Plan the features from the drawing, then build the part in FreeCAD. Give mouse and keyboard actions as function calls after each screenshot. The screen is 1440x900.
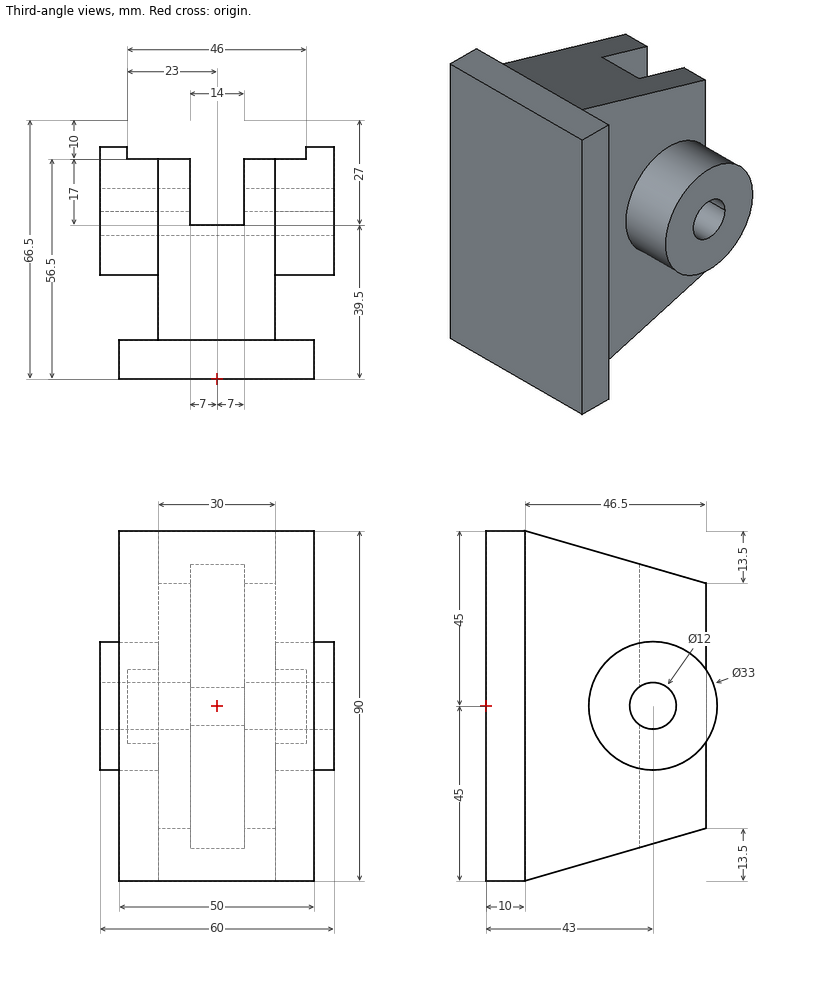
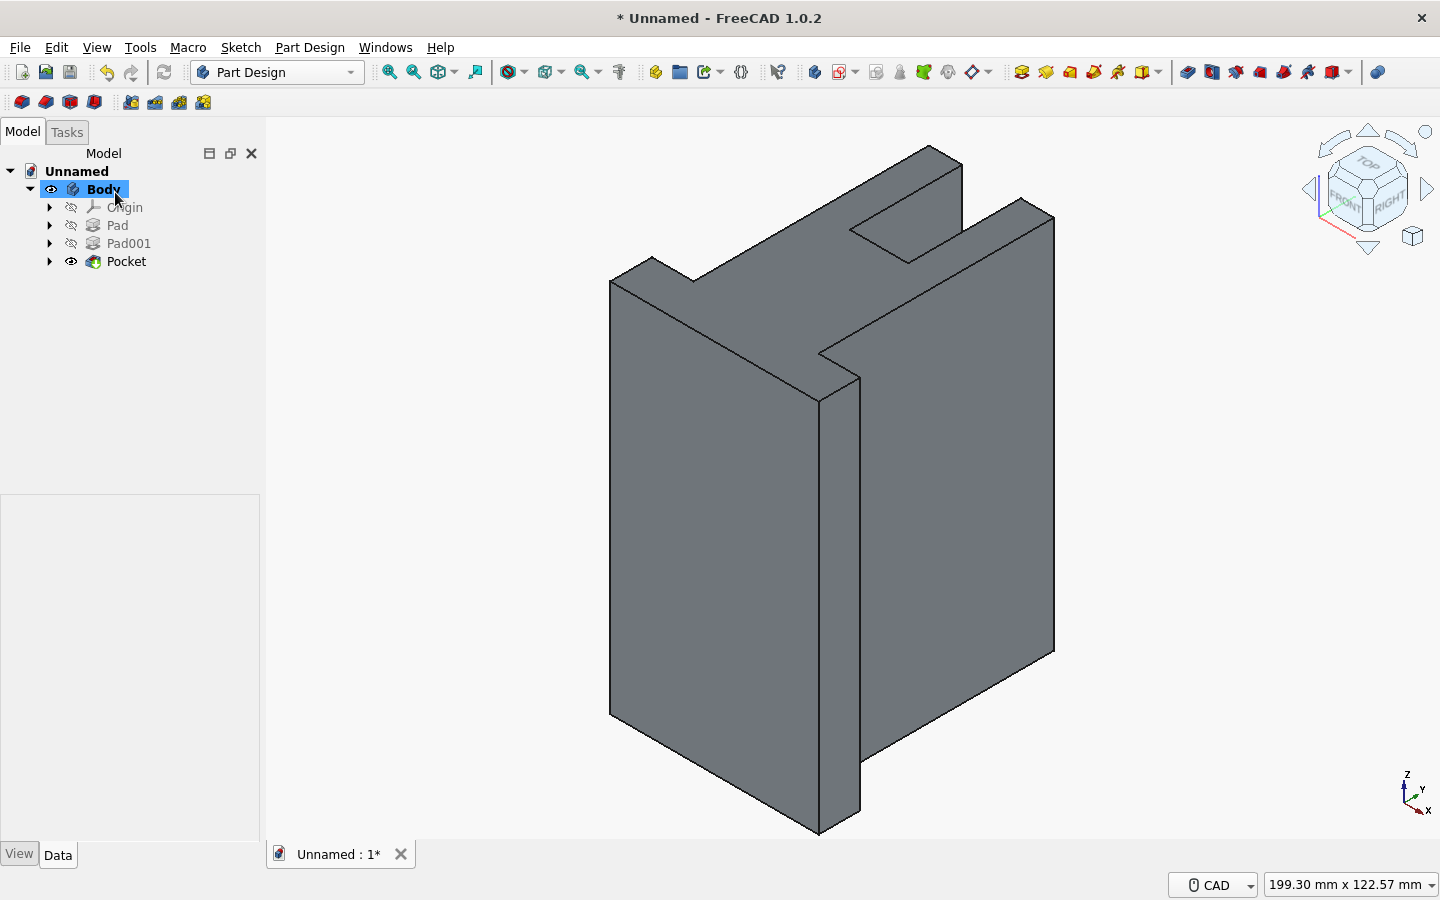
click(840, 72)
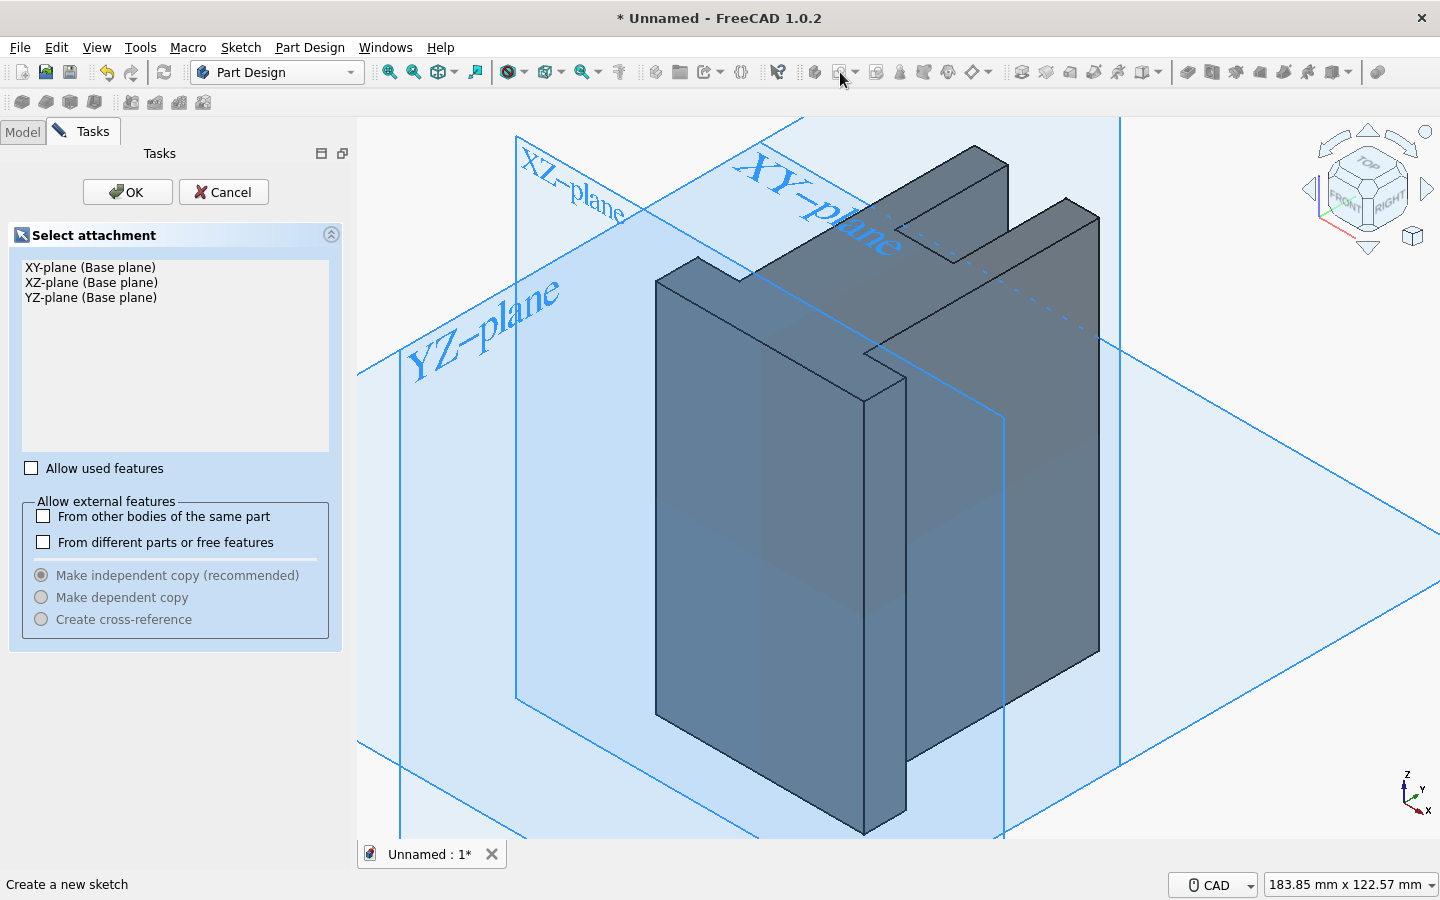
click(82, 298)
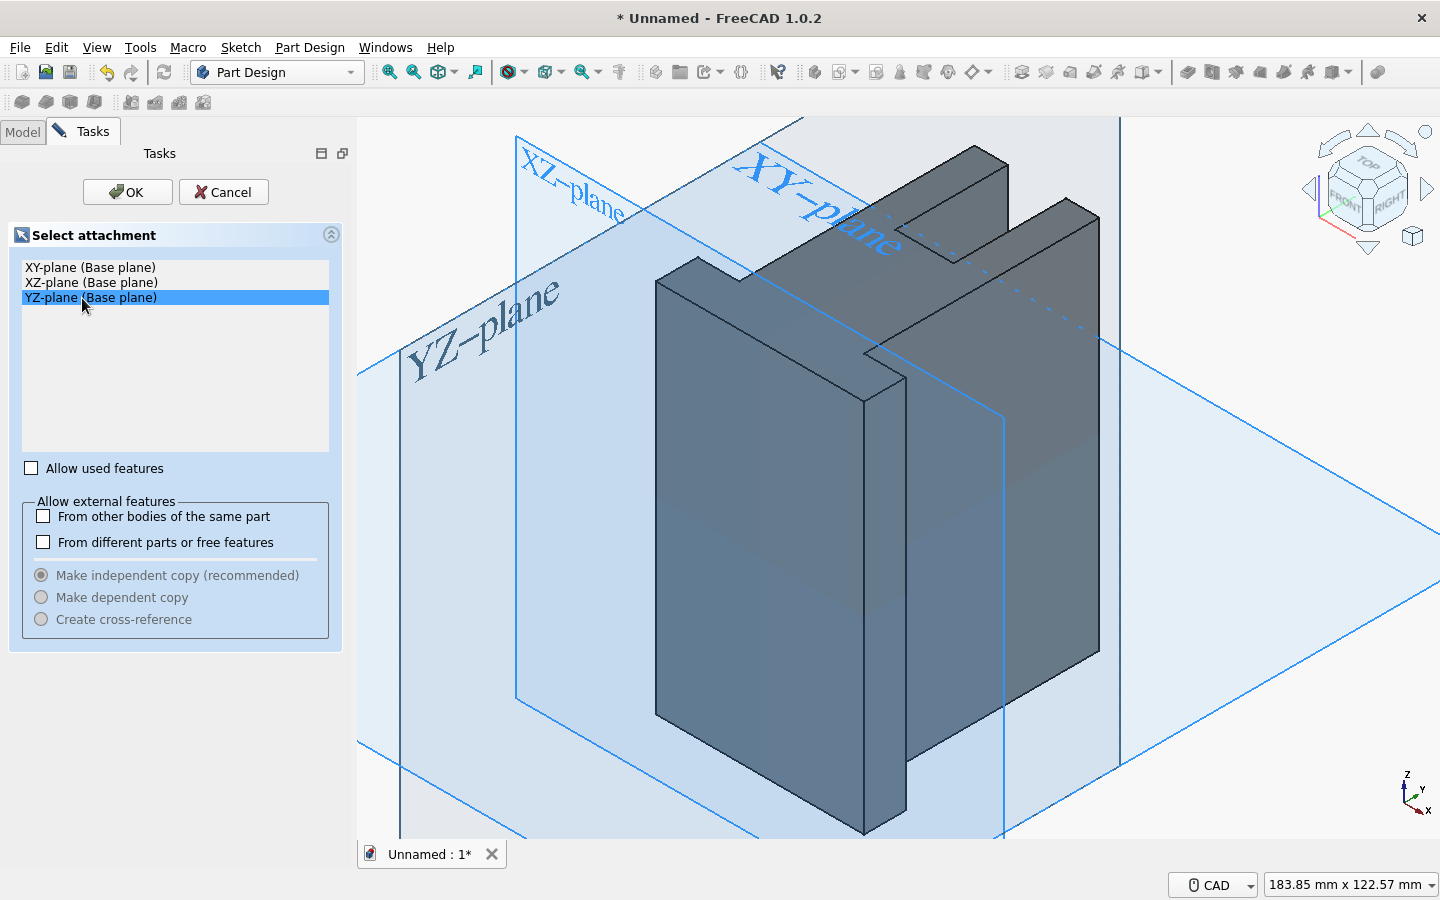
click(128, 192)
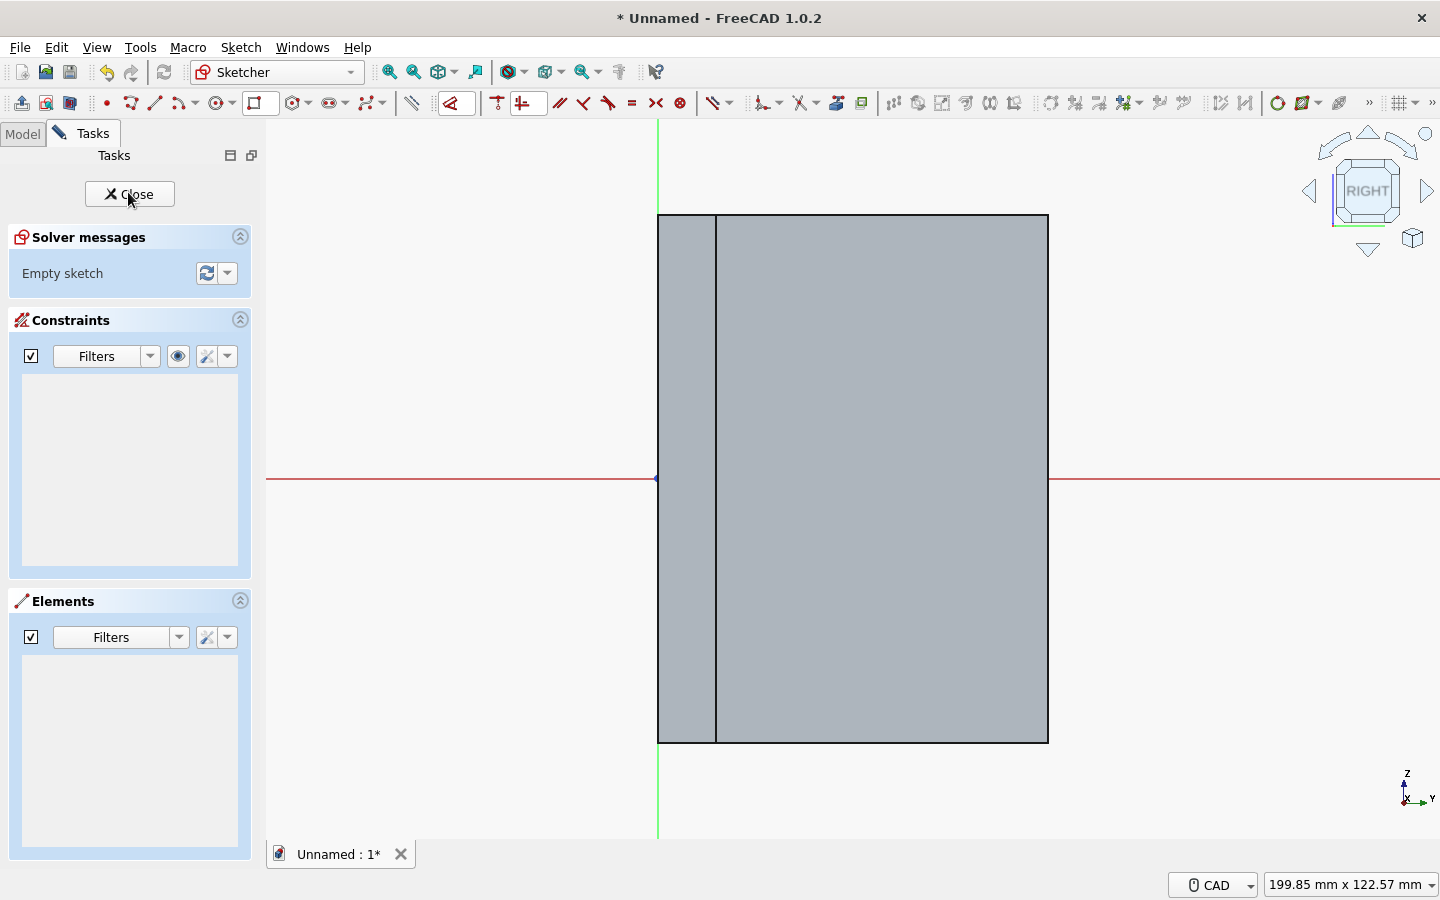
click(70, 104)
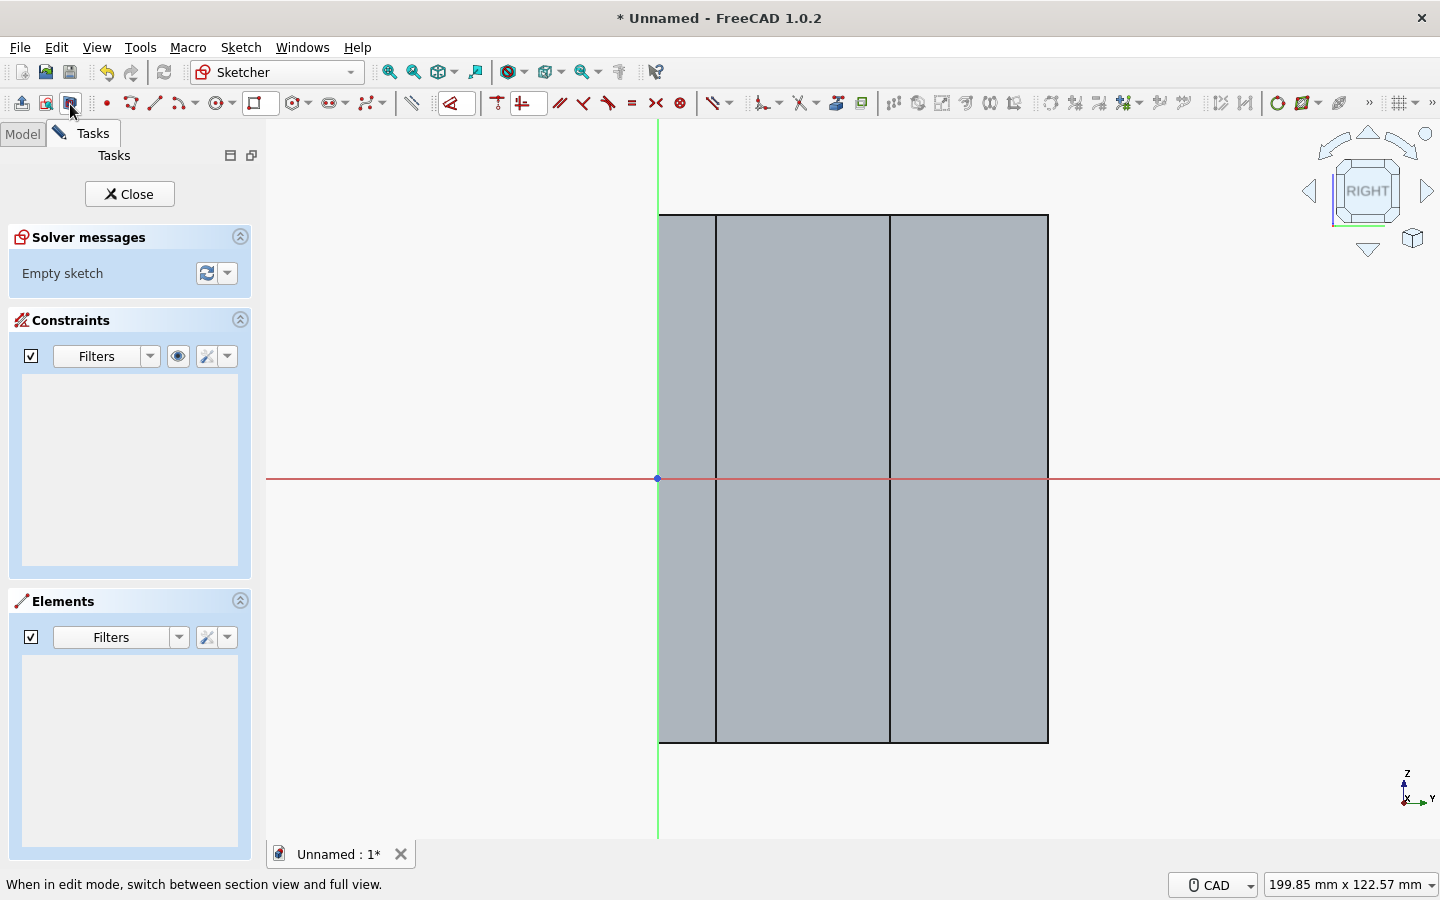
scroll(891, 479, up, 3)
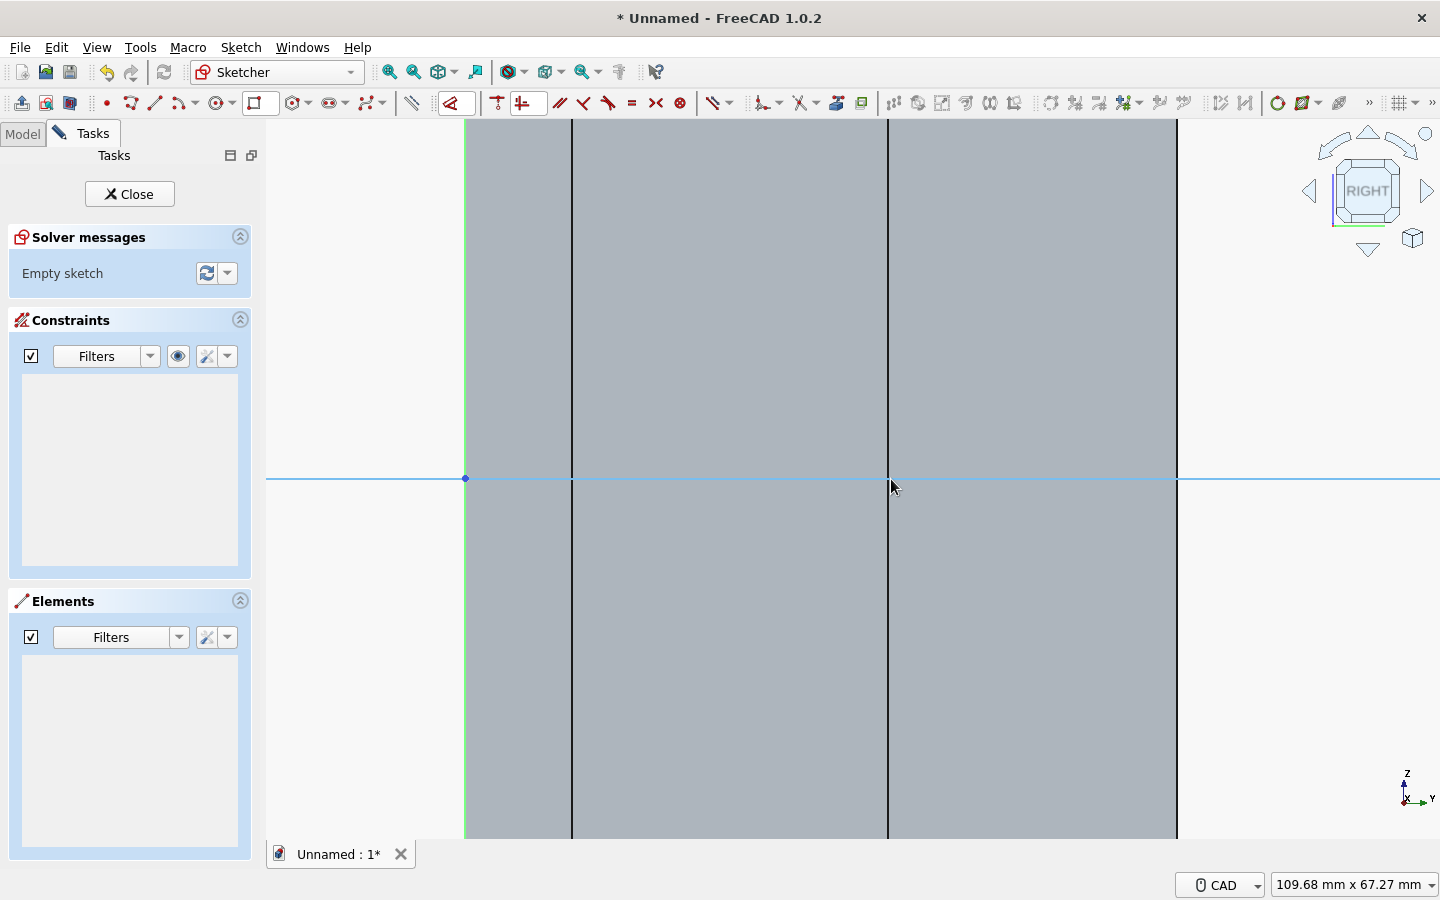
click(216, 104)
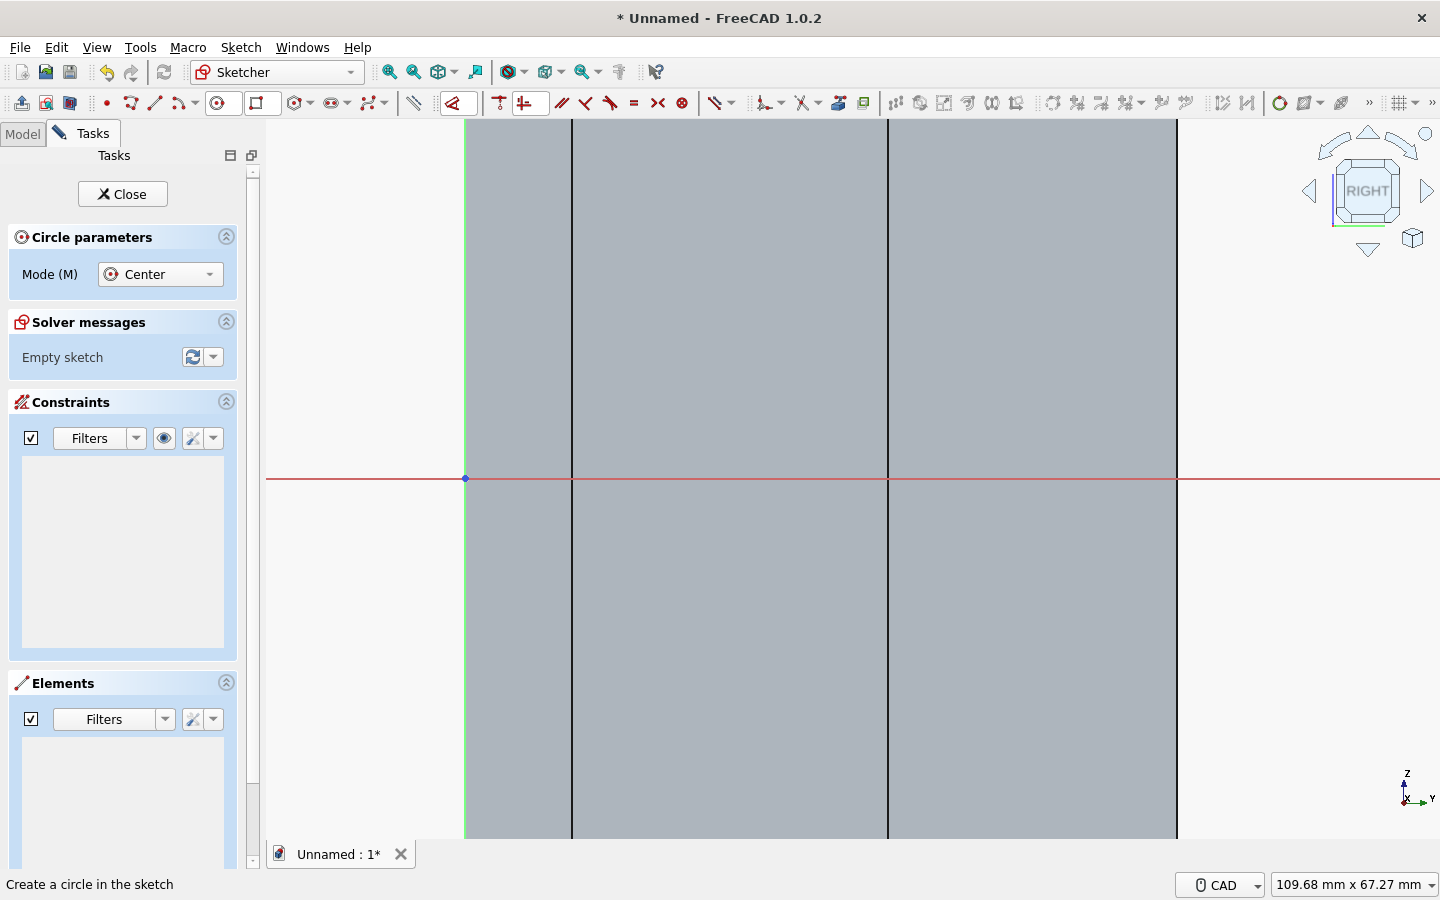
click(926, 479)
click(1051, 354)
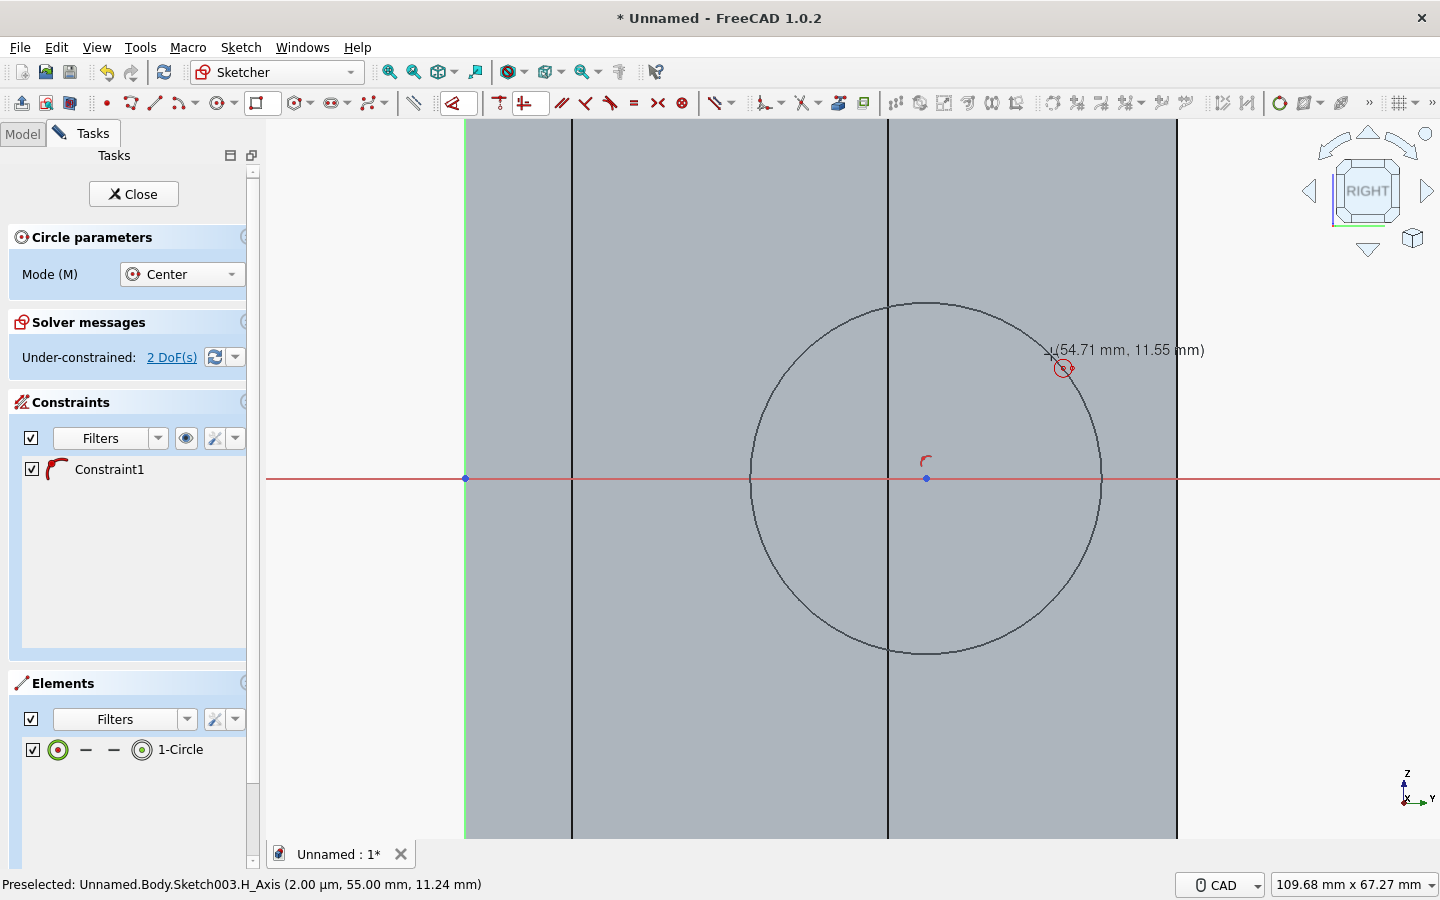
click(926, 479)
click(971, 433)
key(Escape)